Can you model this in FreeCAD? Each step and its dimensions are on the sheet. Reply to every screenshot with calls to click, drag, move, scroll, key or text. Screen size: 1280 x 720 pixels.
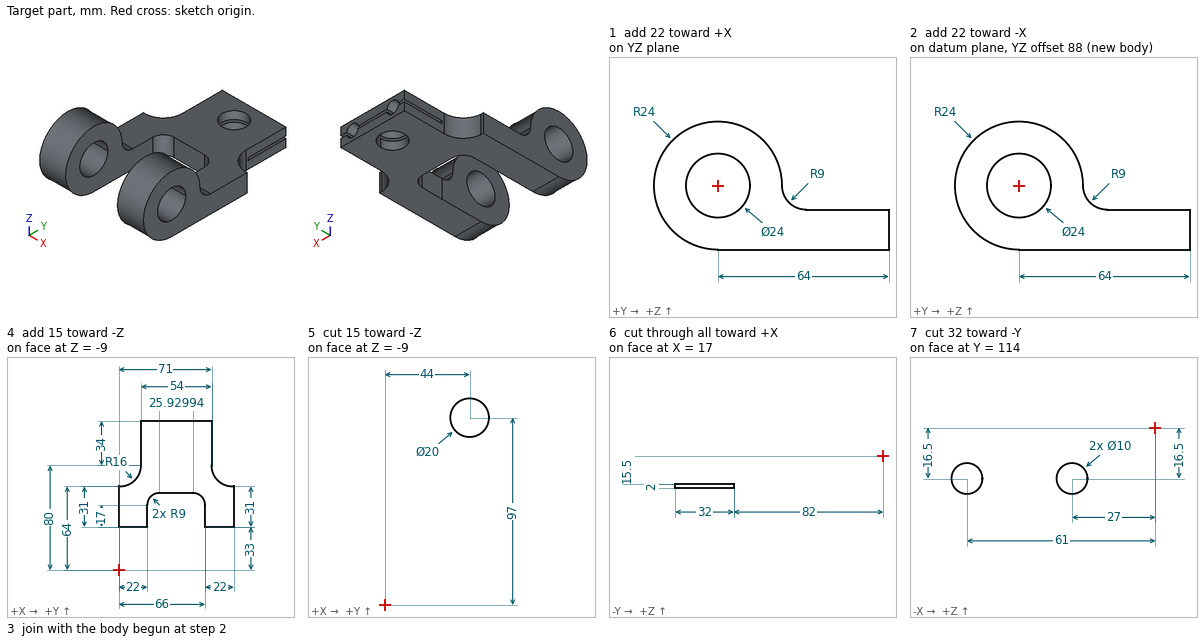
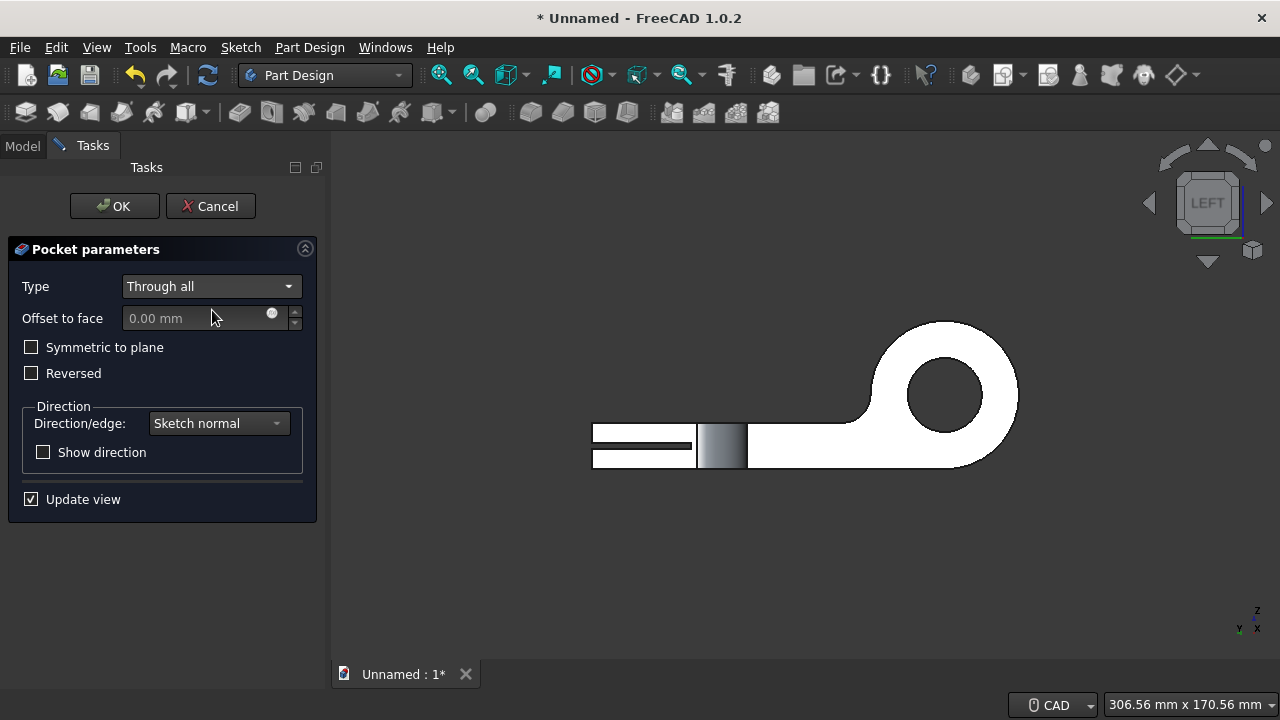
click(115, 206)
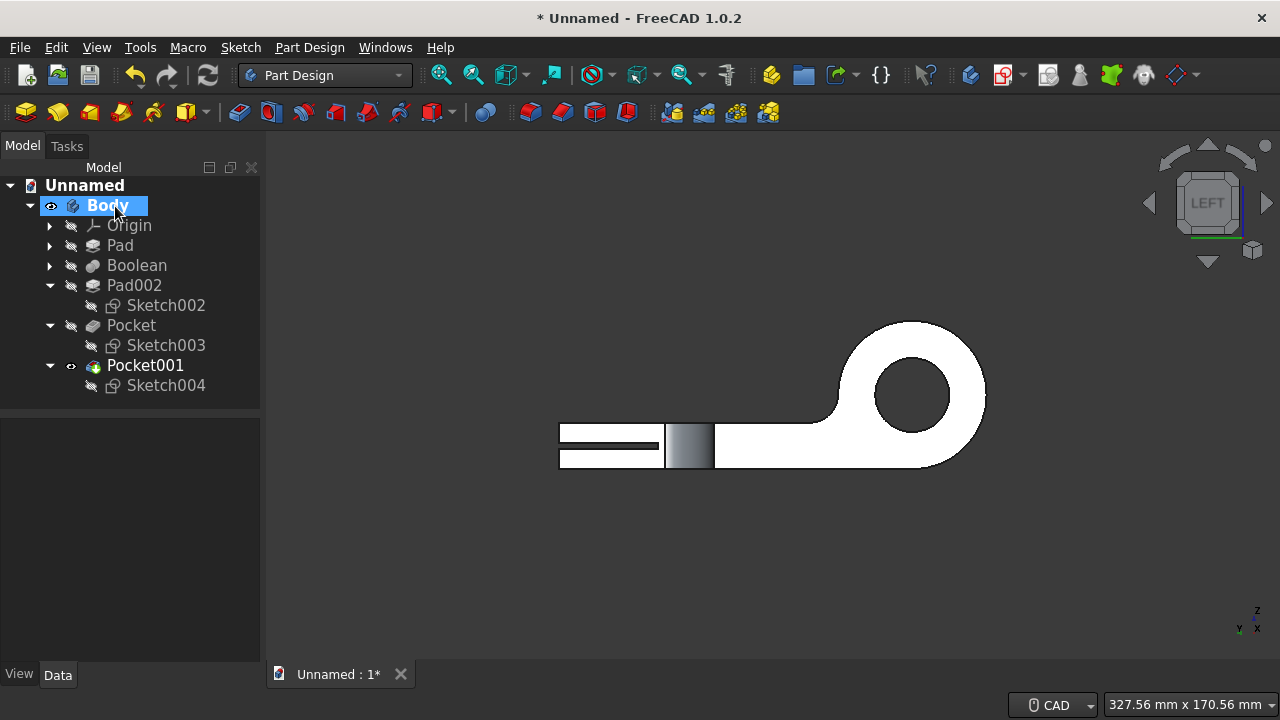
click(442, 76)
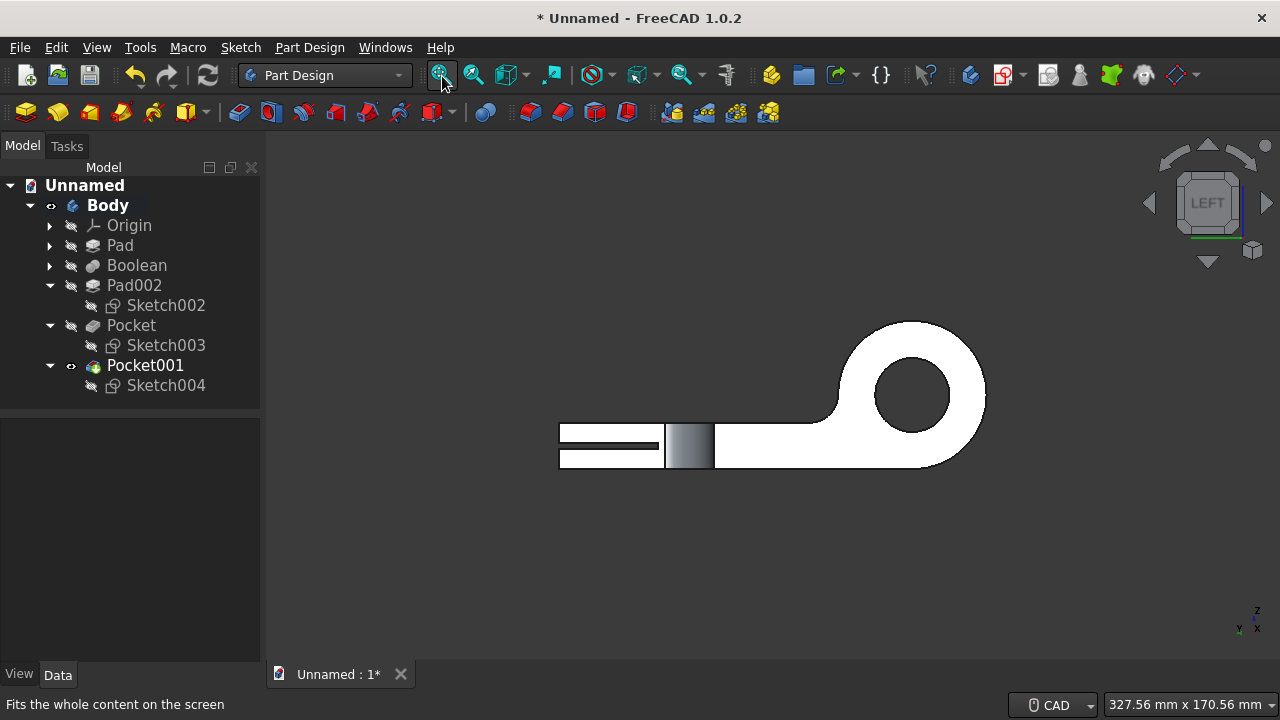
key(4)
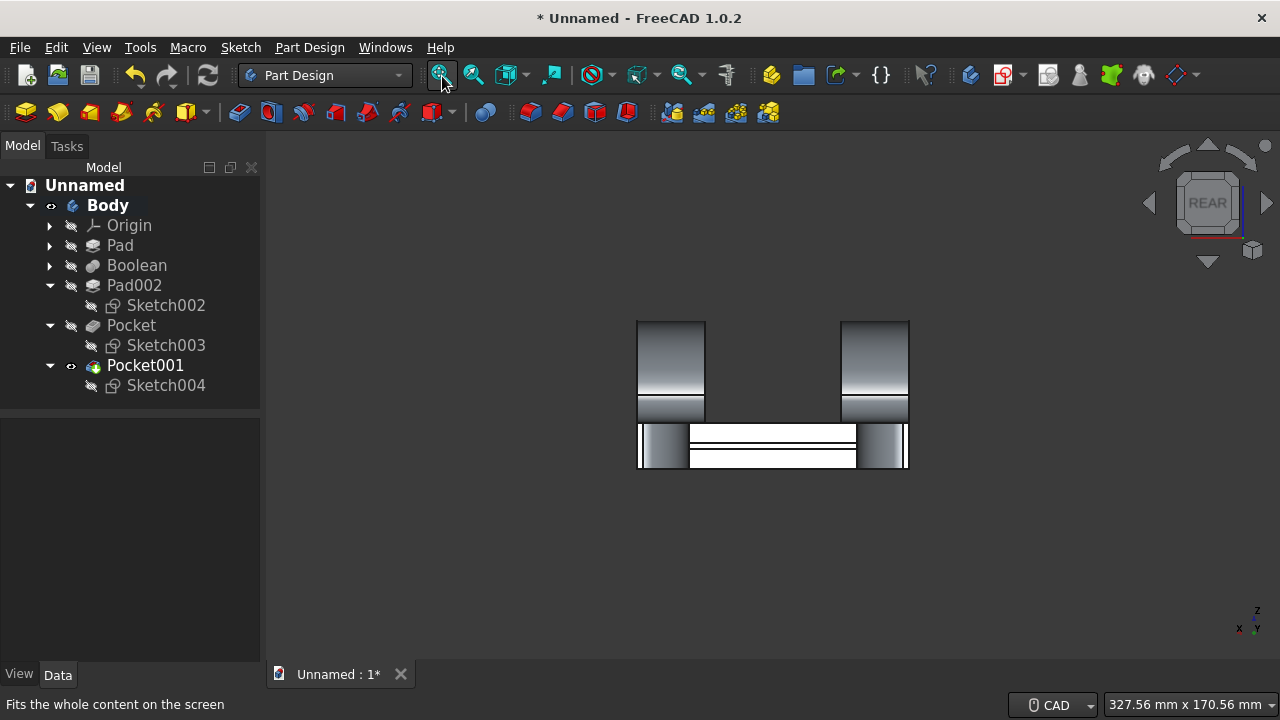
click(442, 76)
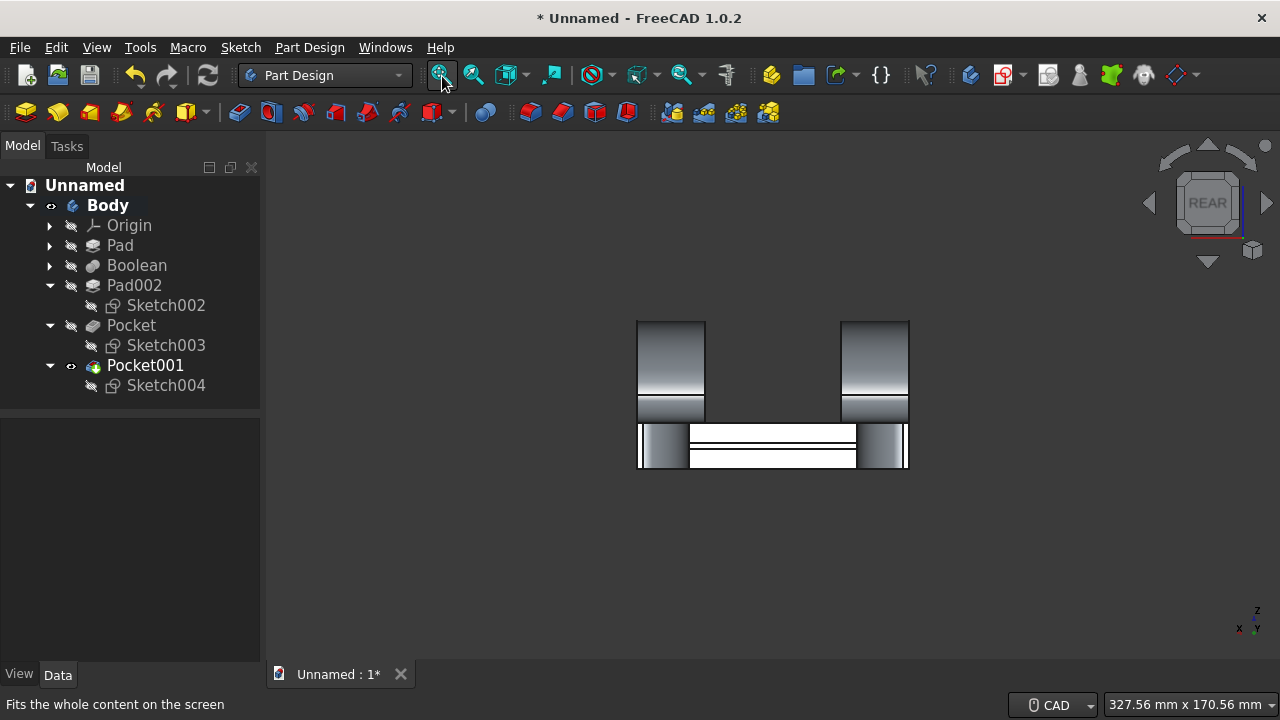
click(701, 458)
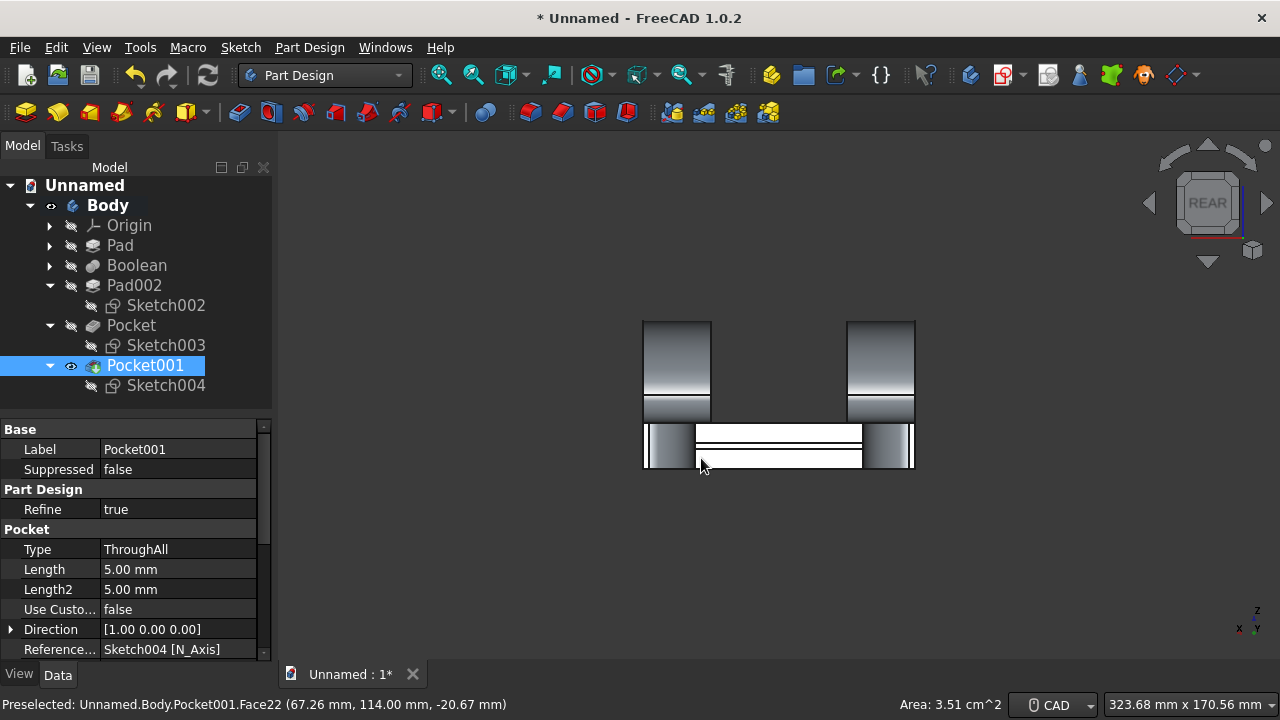
click(1004, 76)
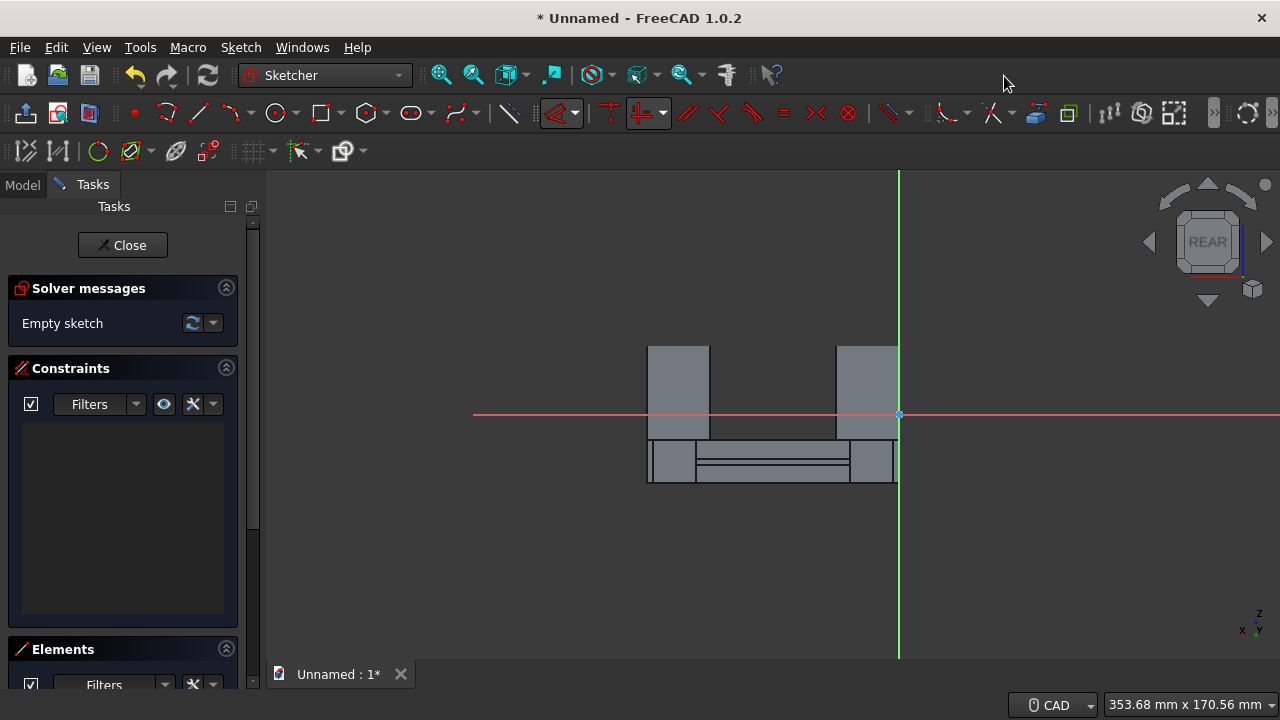
scroll(848, 459, up, 6)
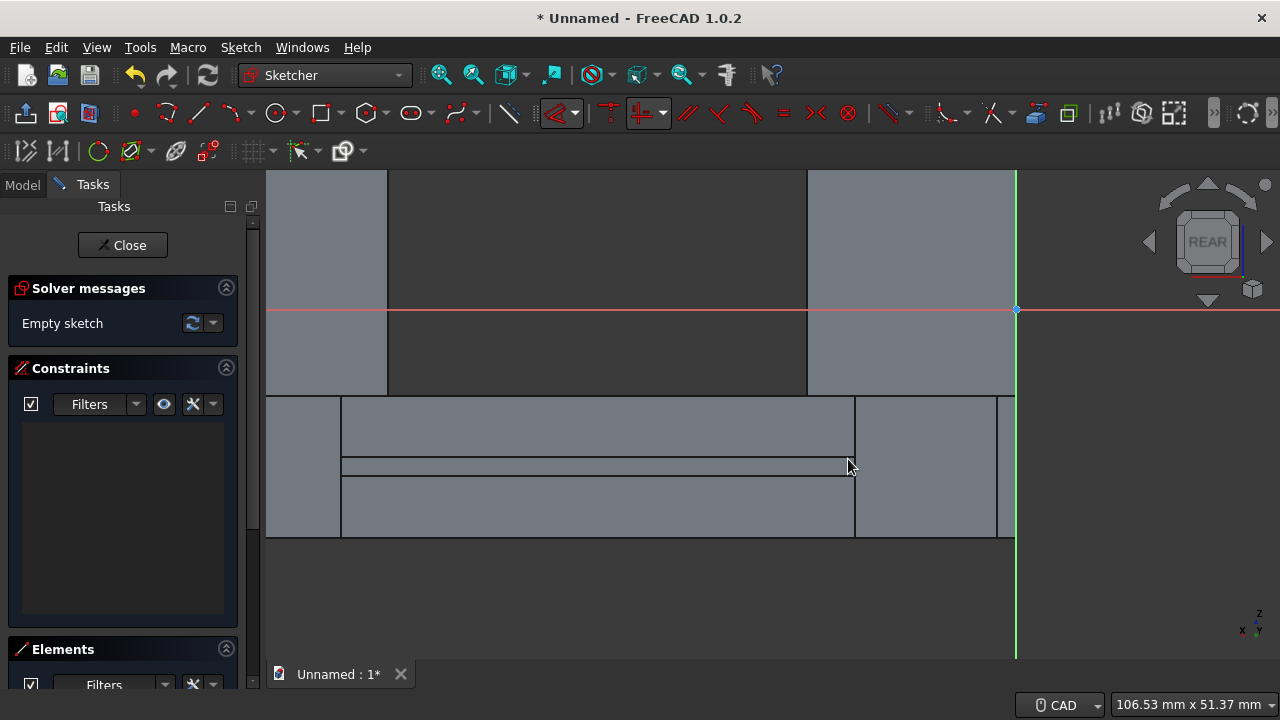
click(276, 114)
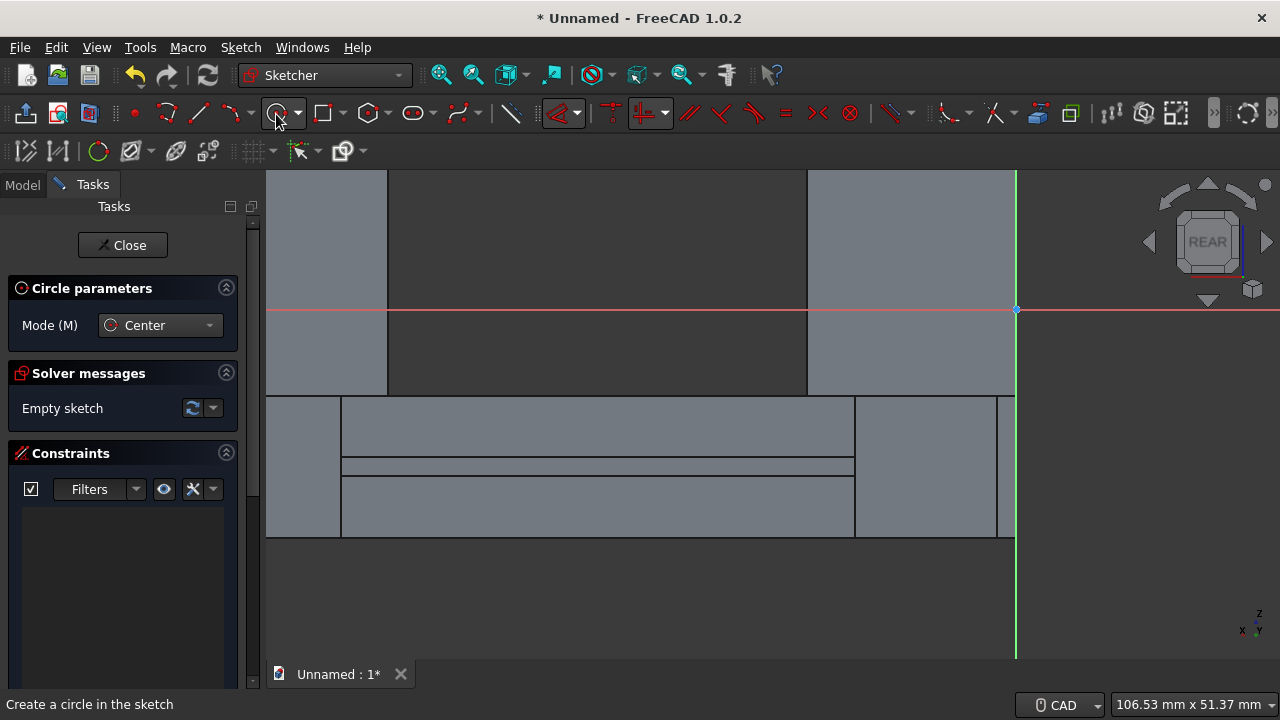
click(759, 467)
click(793, 433)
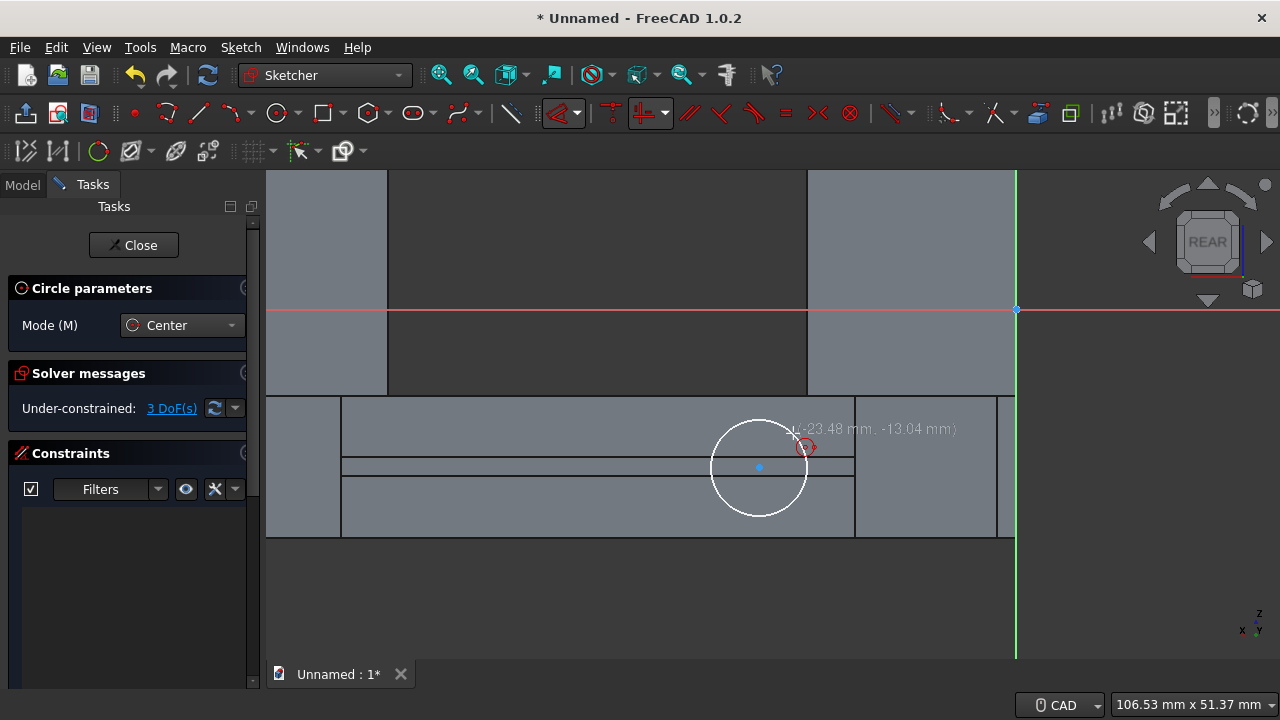
click(436, 467)
click(469, 433)
key(Escape)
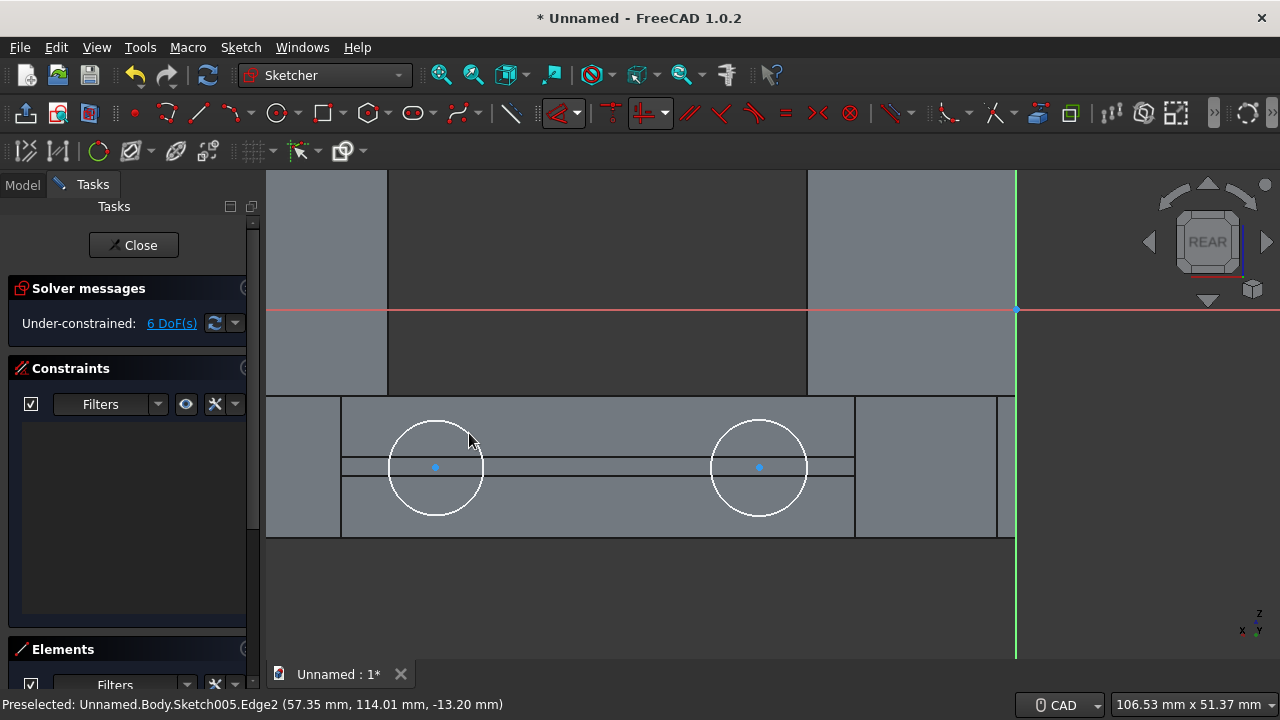
click(793, 434)